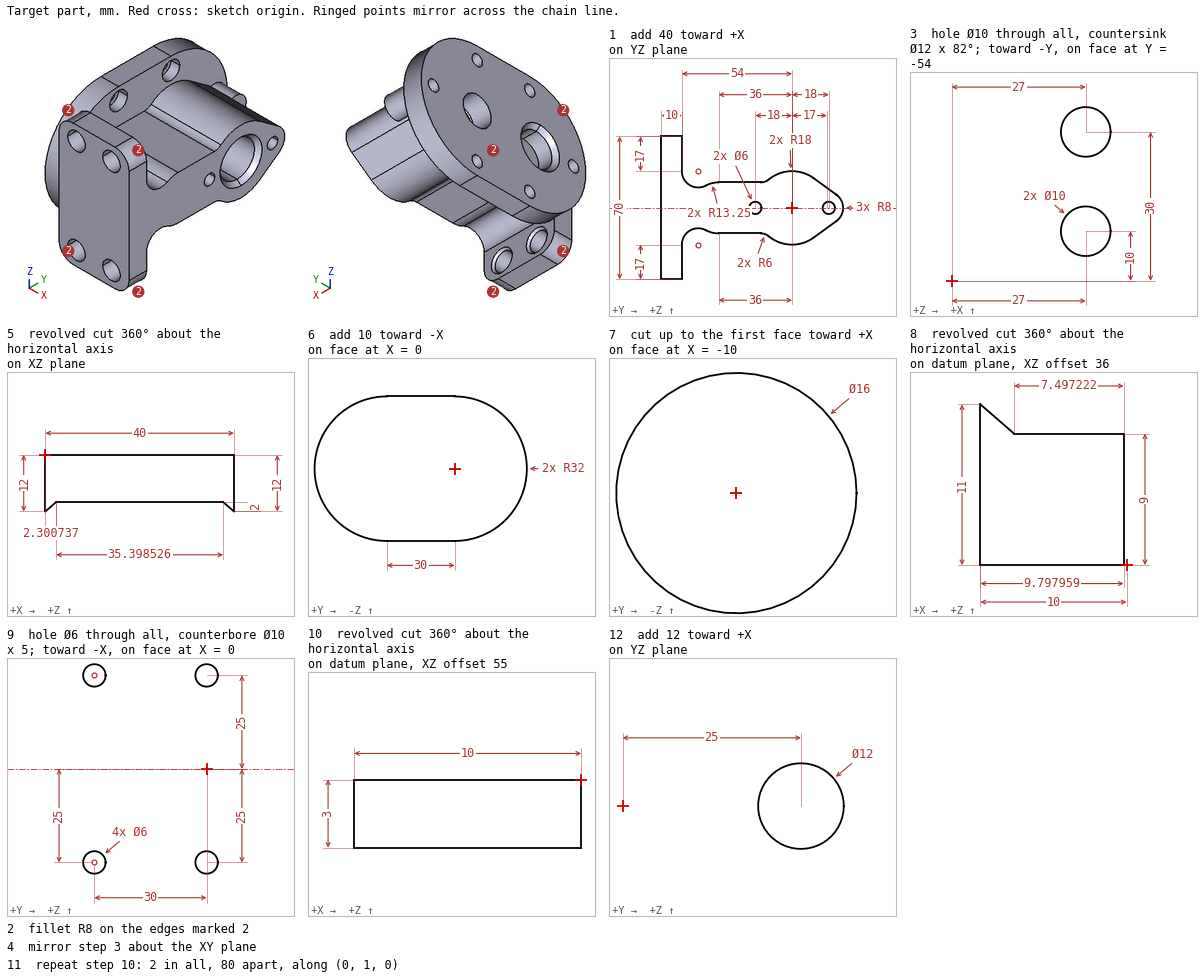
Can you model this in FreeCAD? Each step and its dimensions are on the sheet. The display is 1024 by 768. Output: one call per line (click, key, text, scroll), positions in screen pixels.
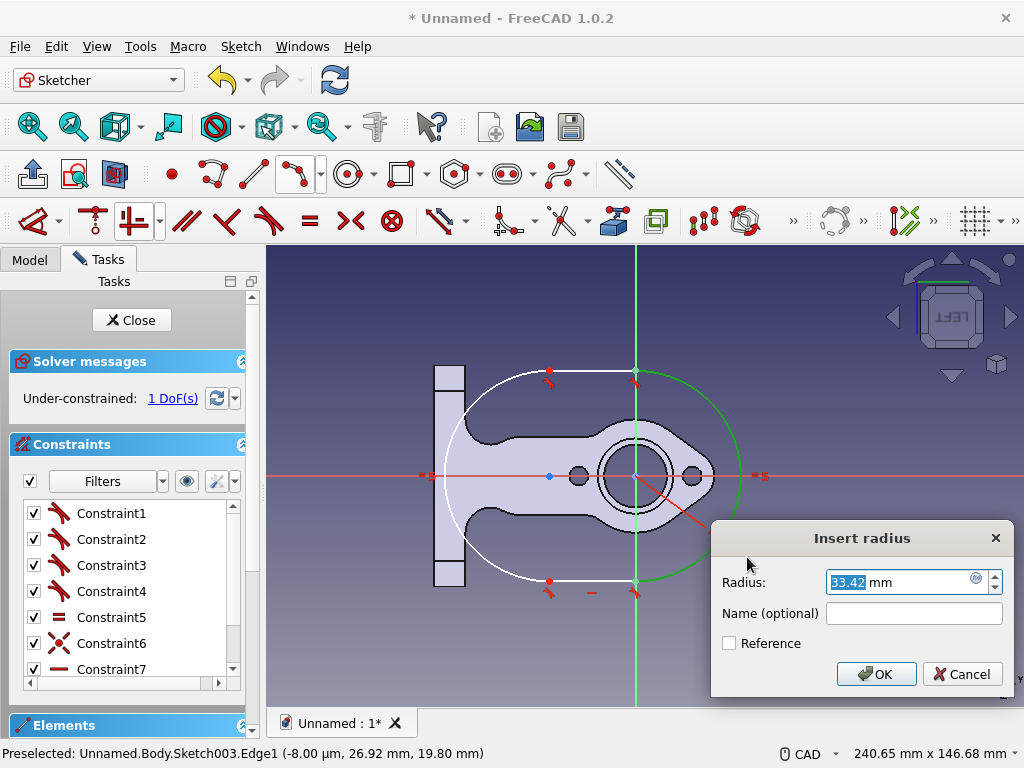
text(32)
key(Return)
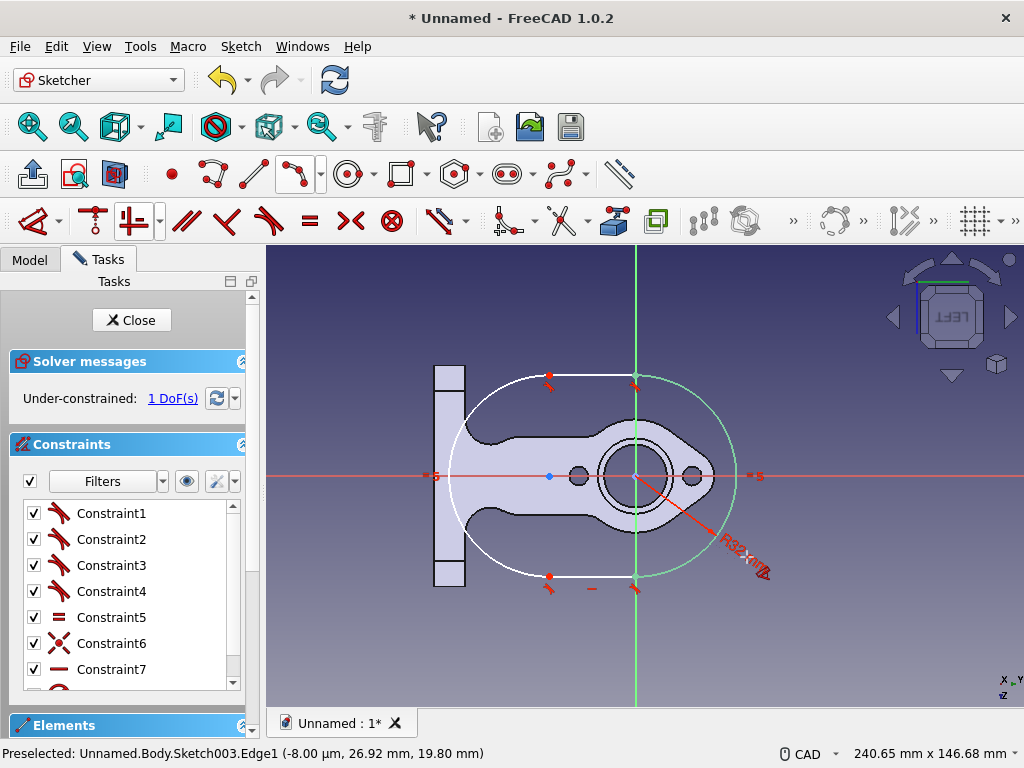
click(610, 577)
click(593, 611)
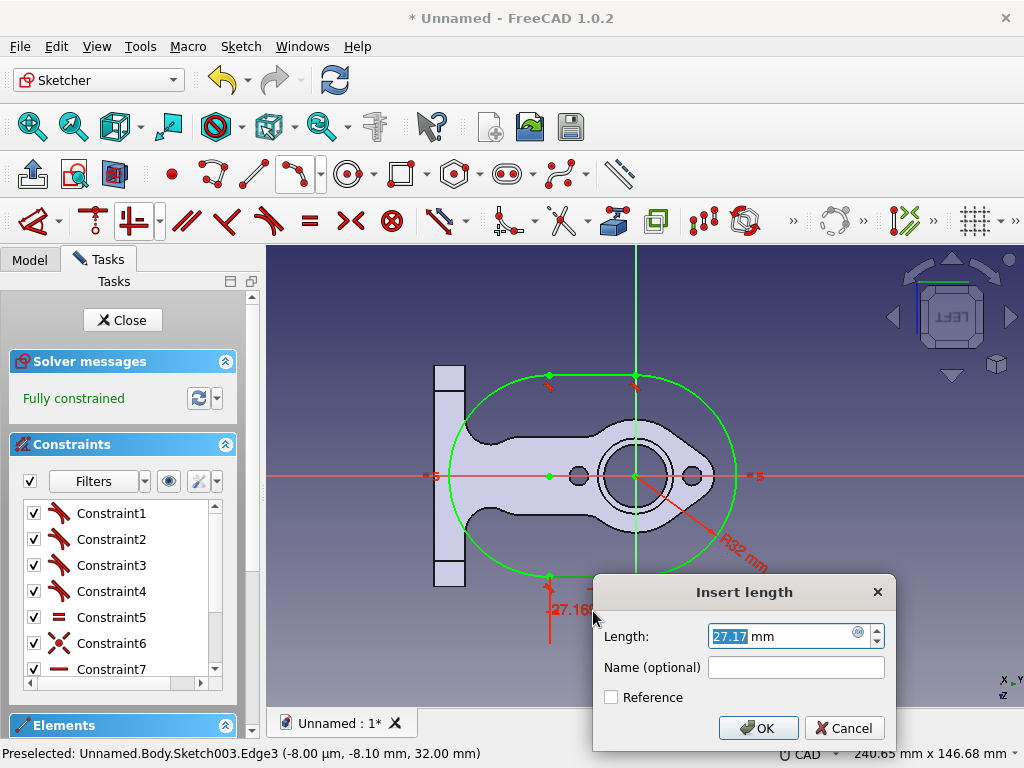
text(30)
key(Return)
key(Escape)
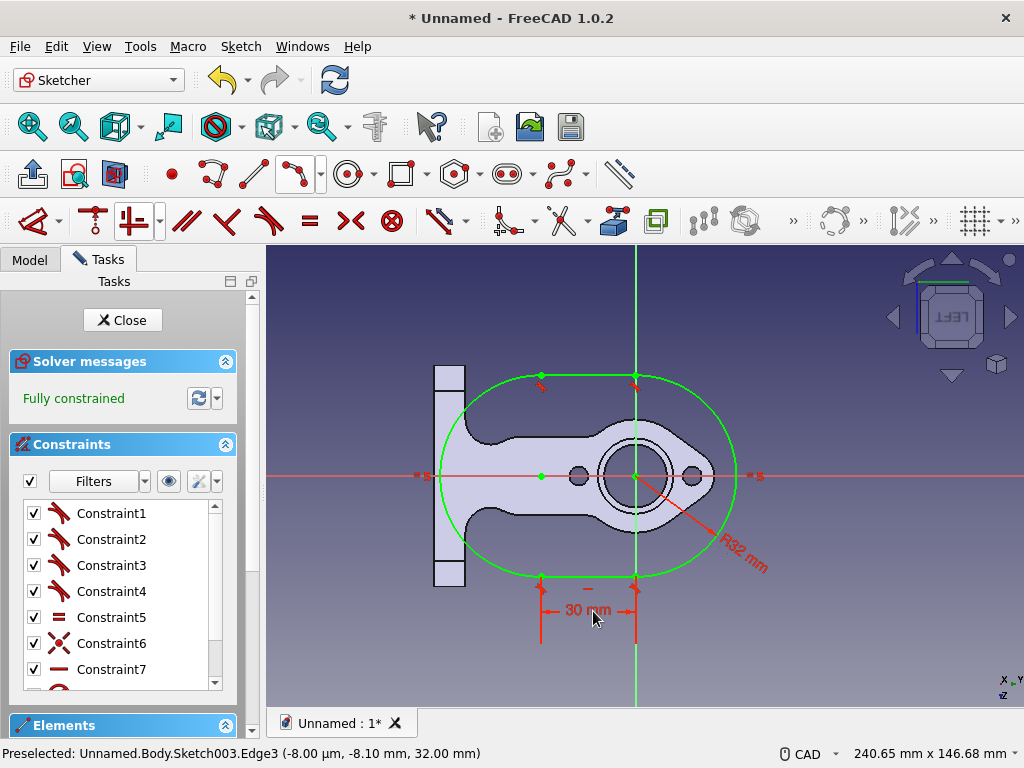
click(123, 320)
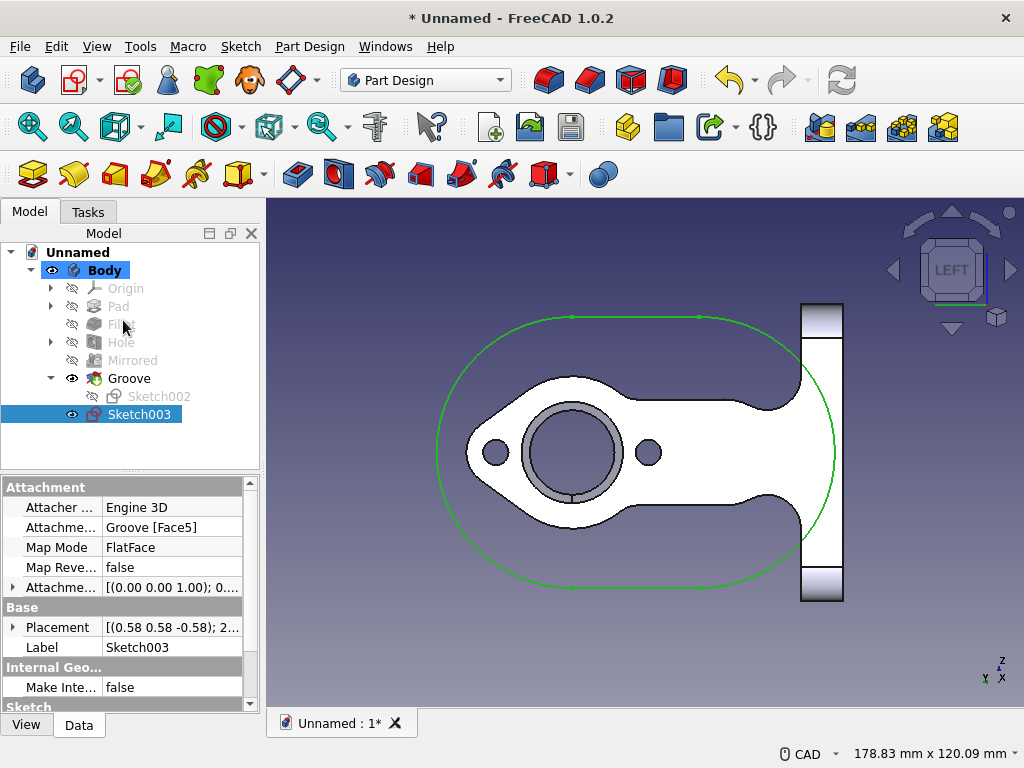
click(33, 174)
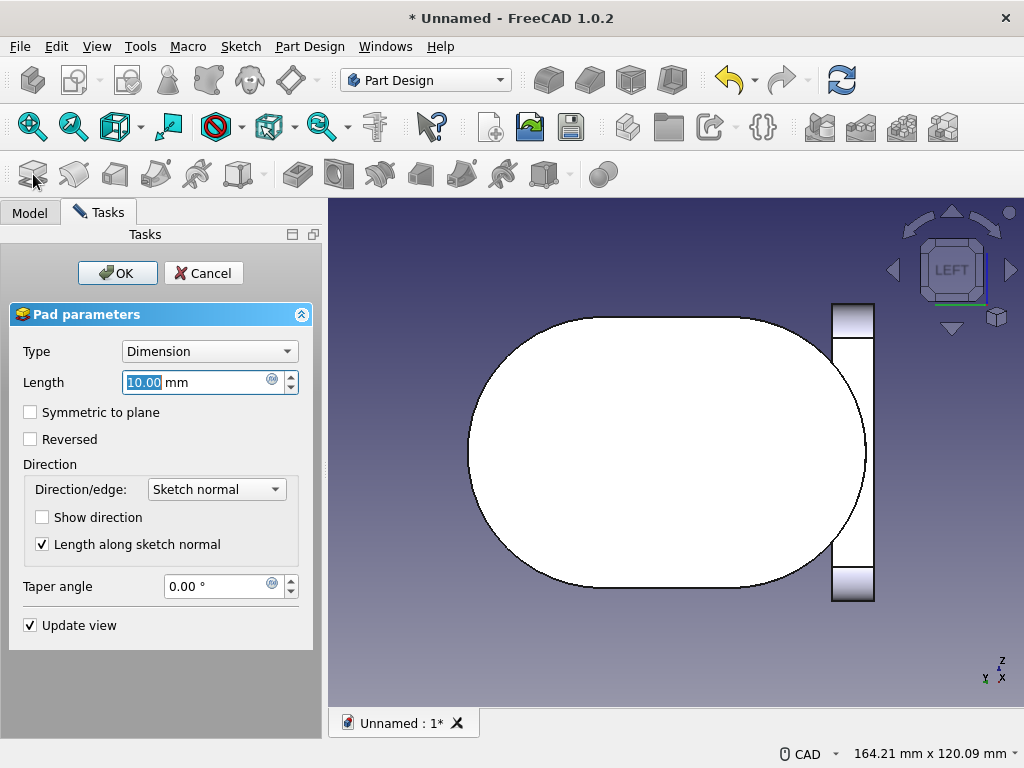
text(10)
key(Tab)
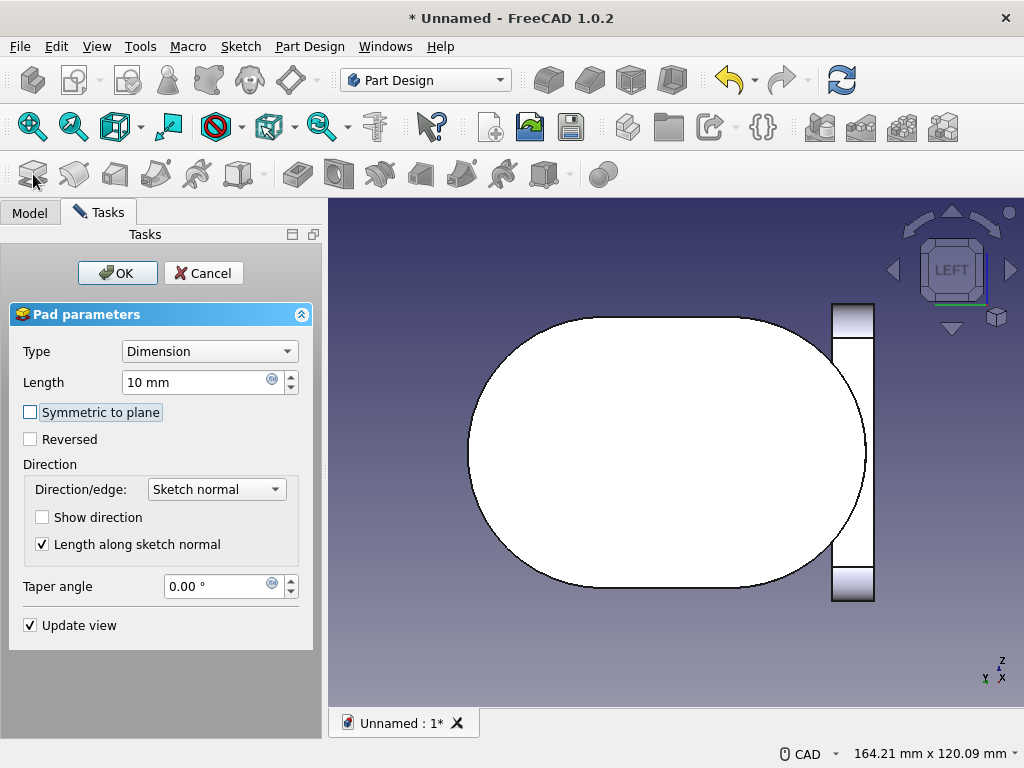
click(118, 273)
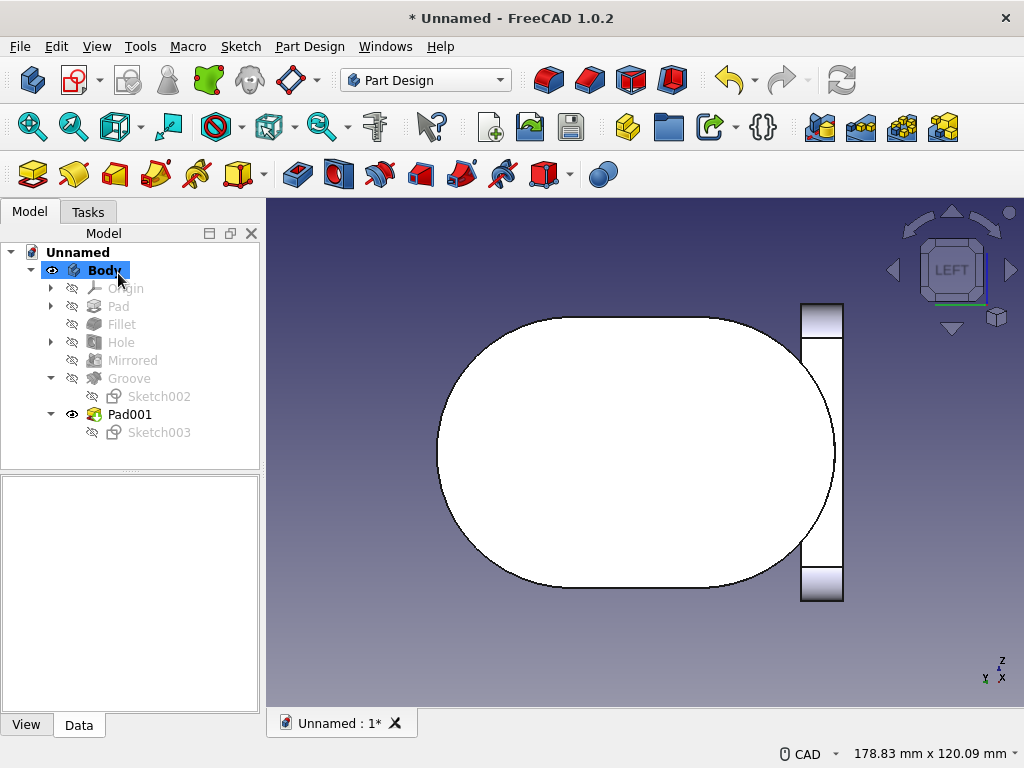
click(579, 451)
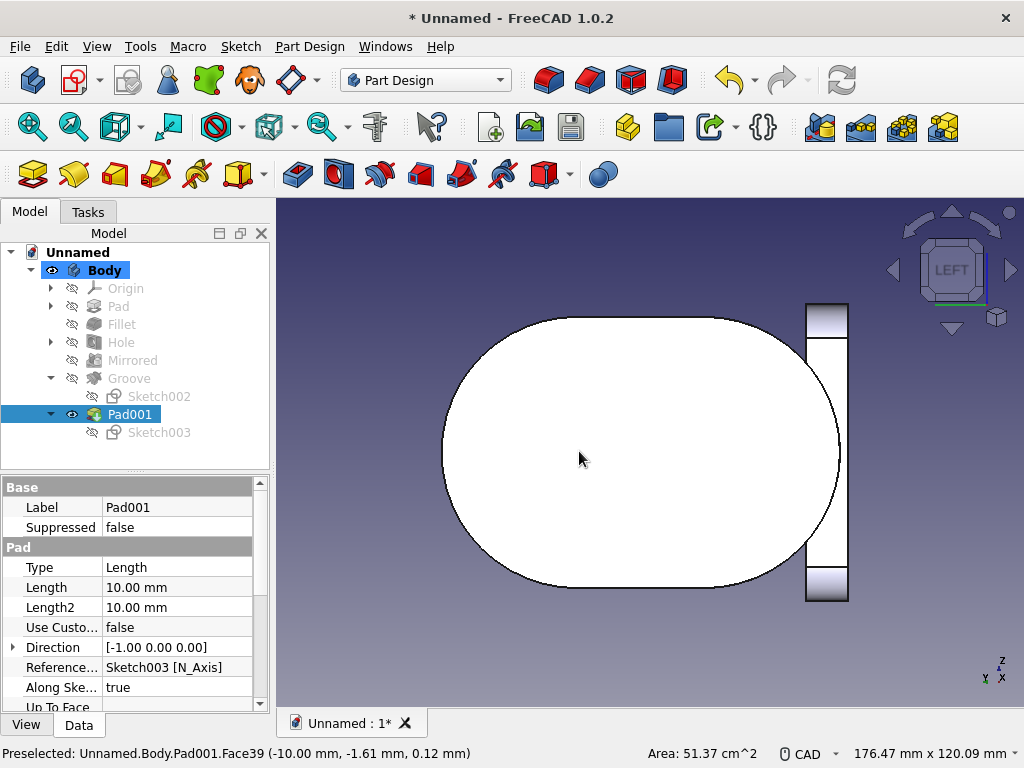
click(74, 80)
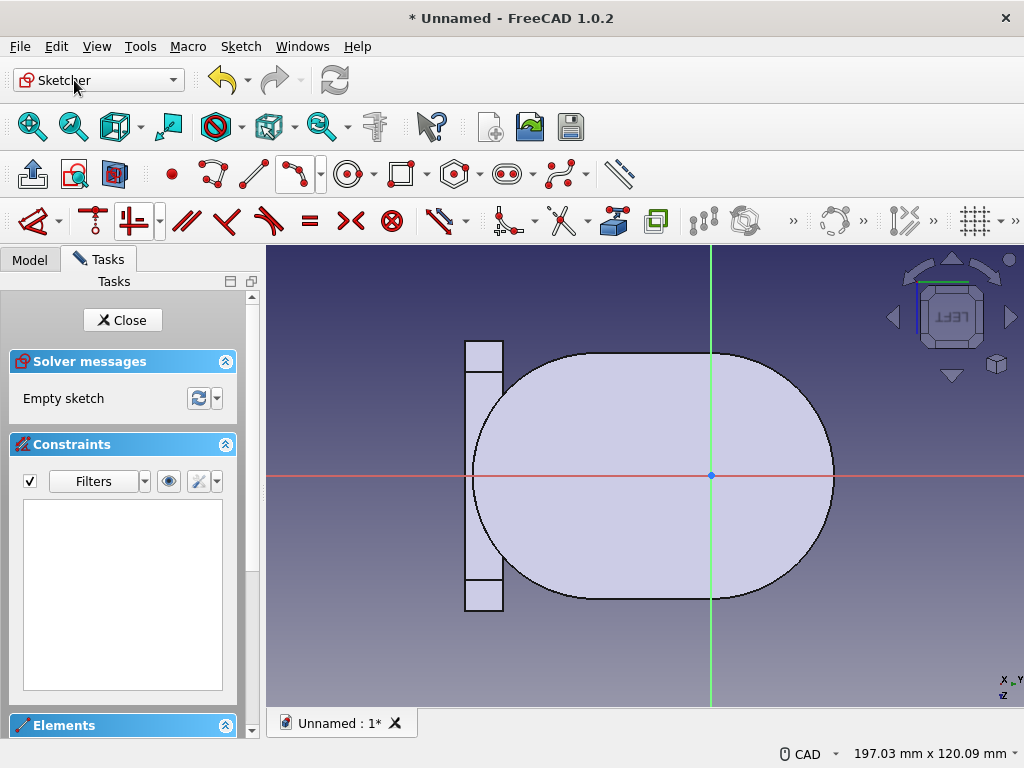
scroll(745, 476, up, 8)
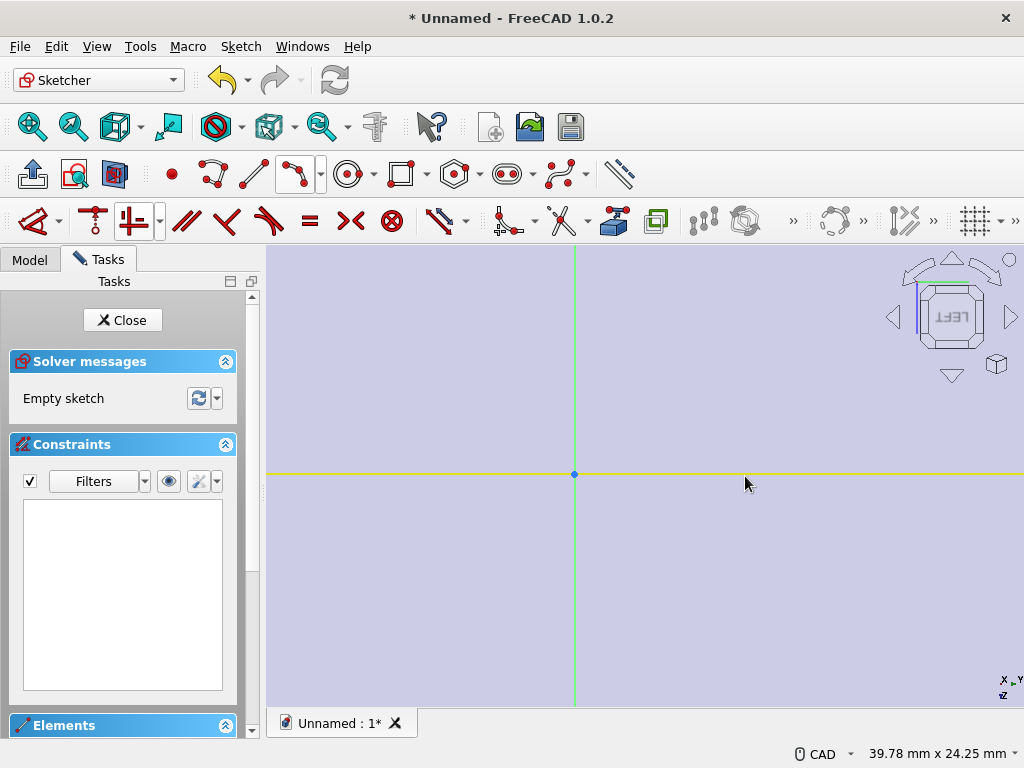
click(348, 174)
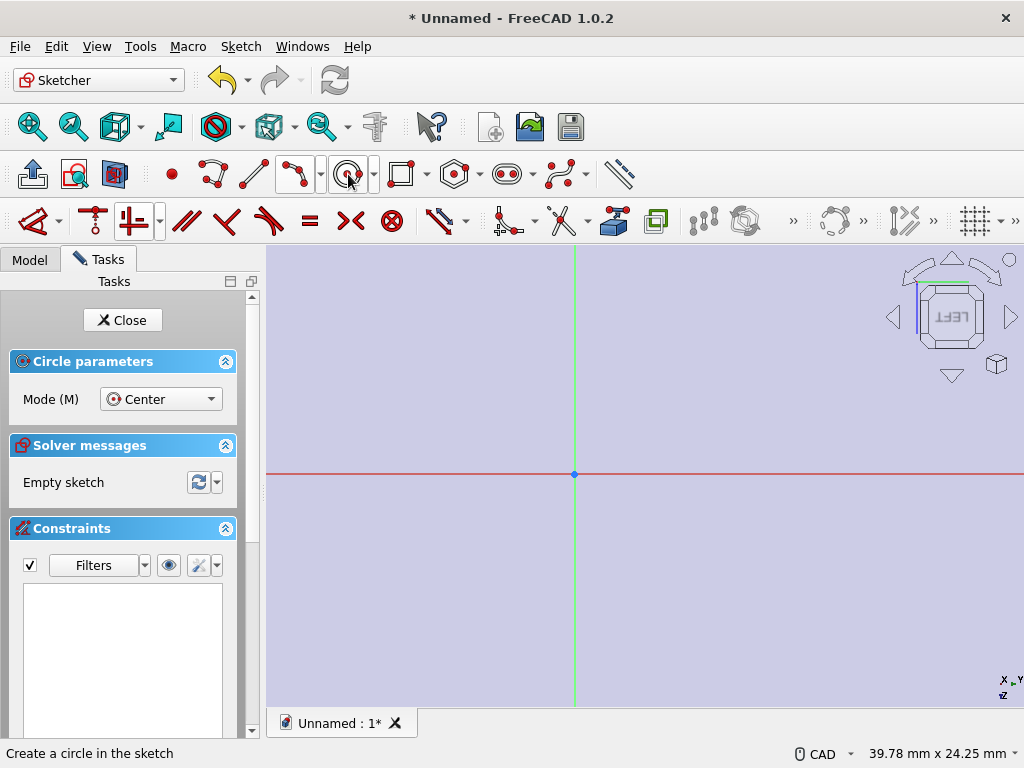
click(575, 474)
click(682, 366)
key(Escape)